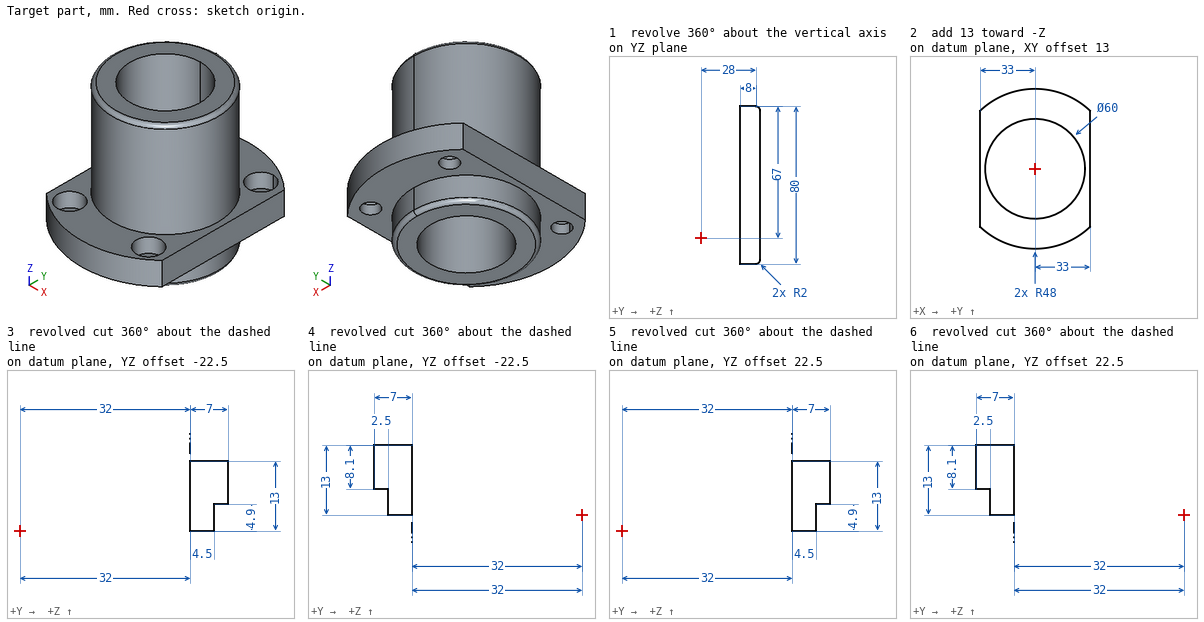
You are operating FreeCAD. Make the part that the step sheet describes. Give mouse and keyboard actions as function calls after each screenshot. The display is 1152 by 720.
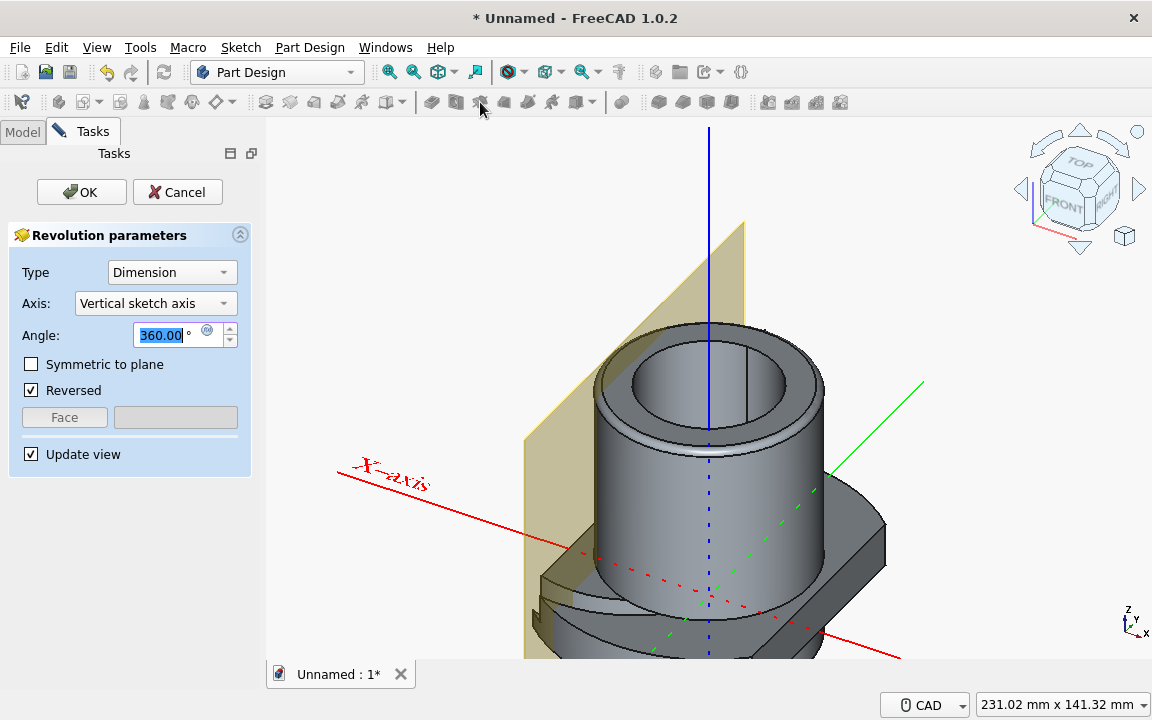
click(156, 304)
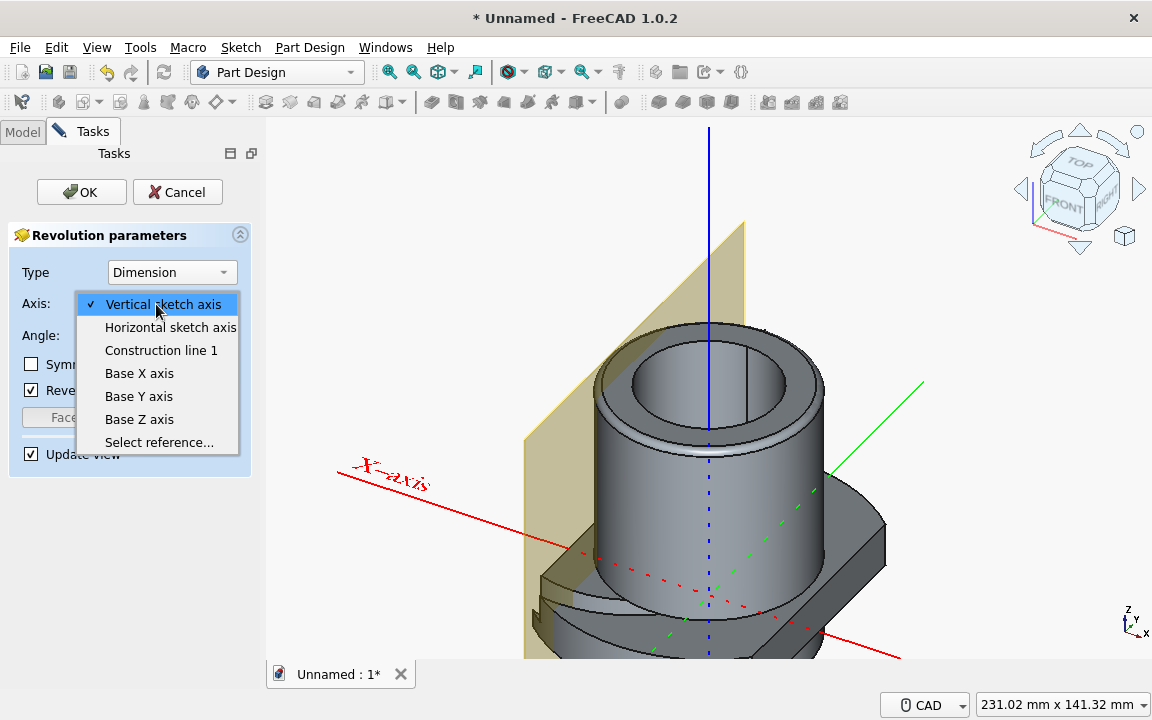
click(156, 350)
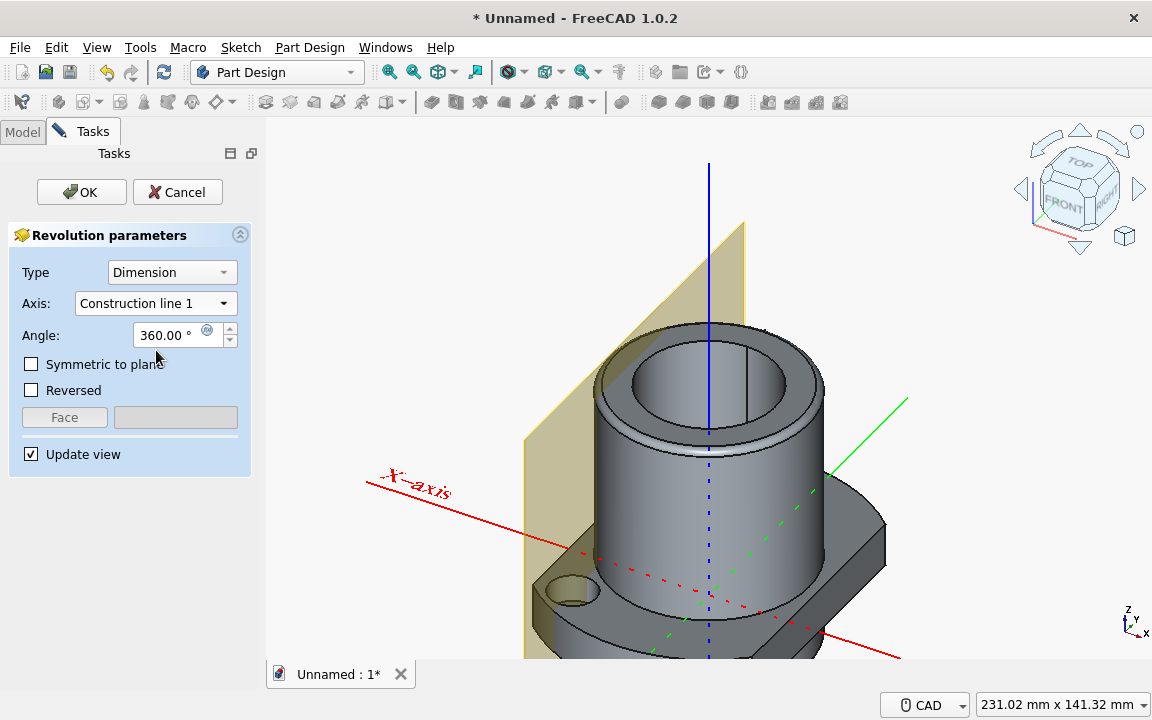
click(82, 192)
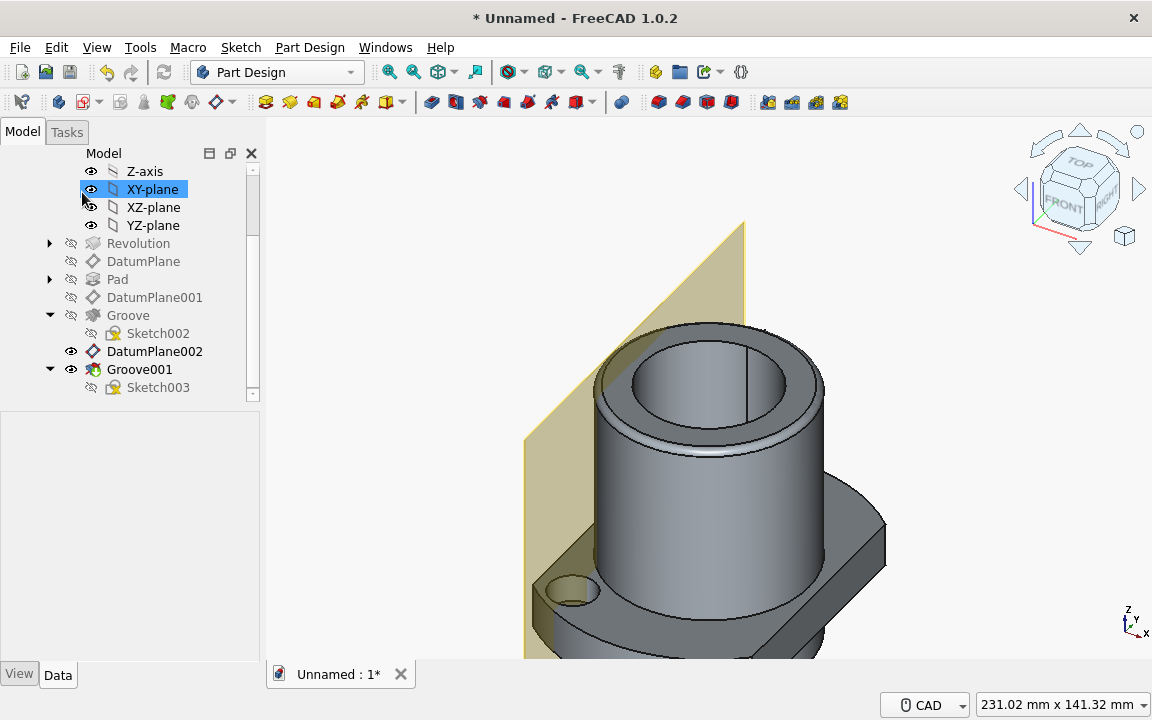
click(116, 351)
key(space)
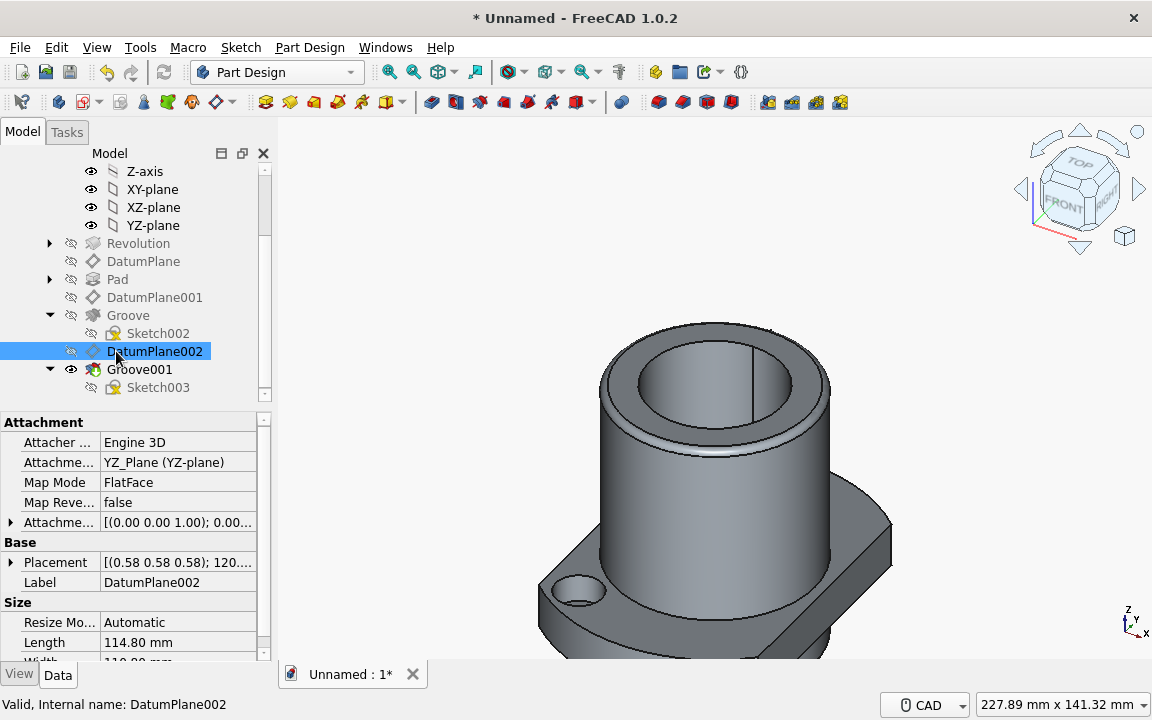
click(390, 72)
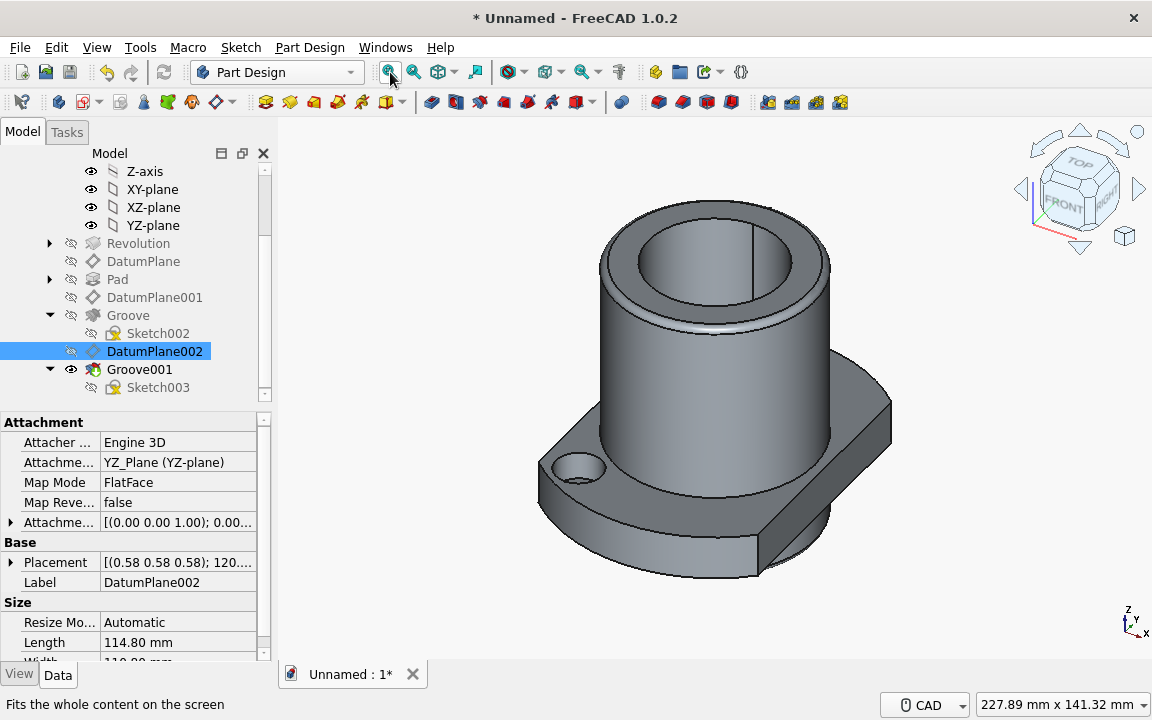
scroll(160, 275, down, 3)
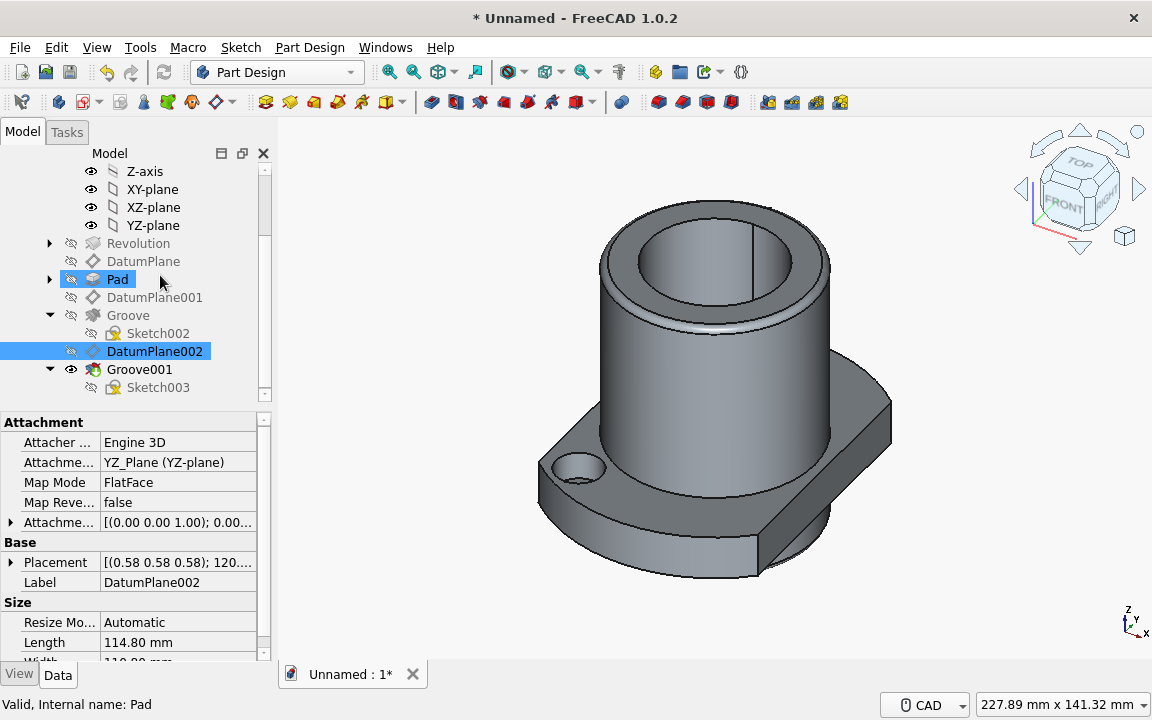
scroll(160, 275, up, 15)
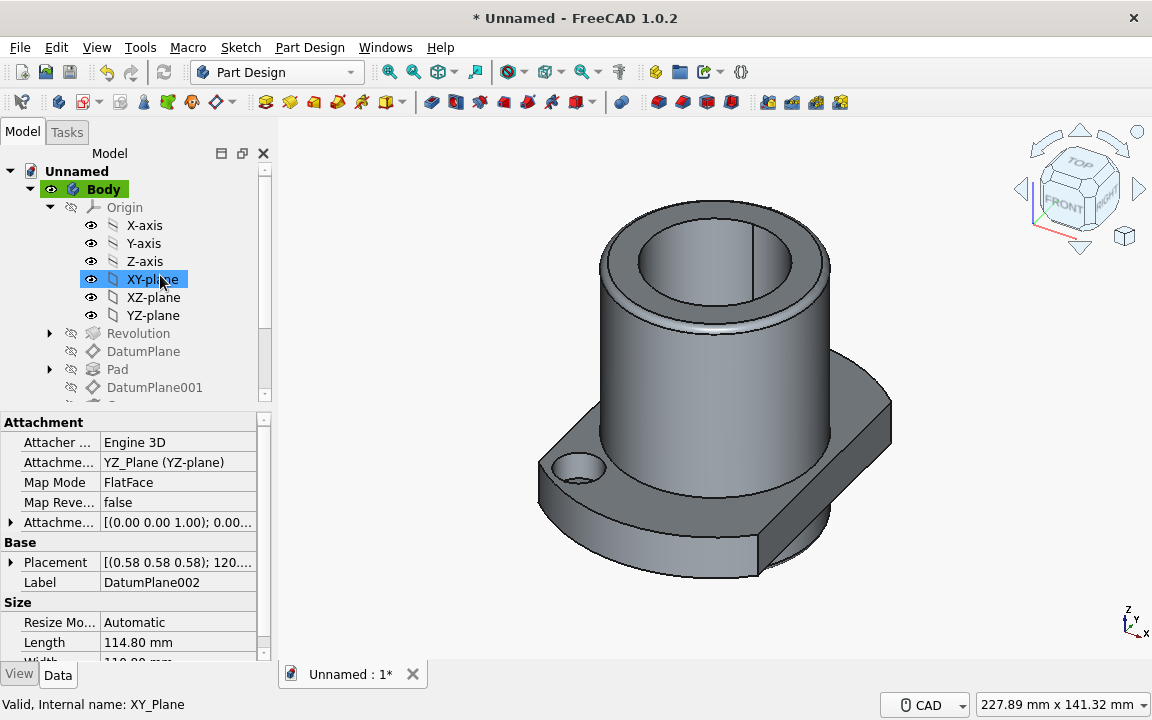
click(136, 315)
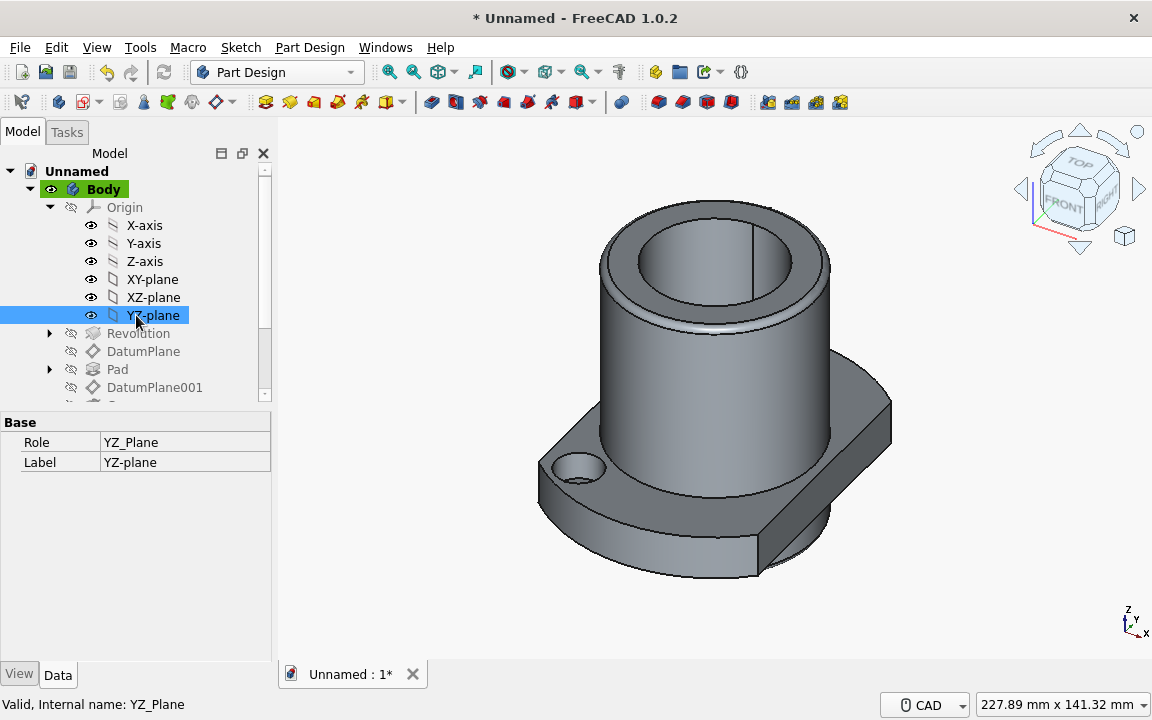
click(216, 102)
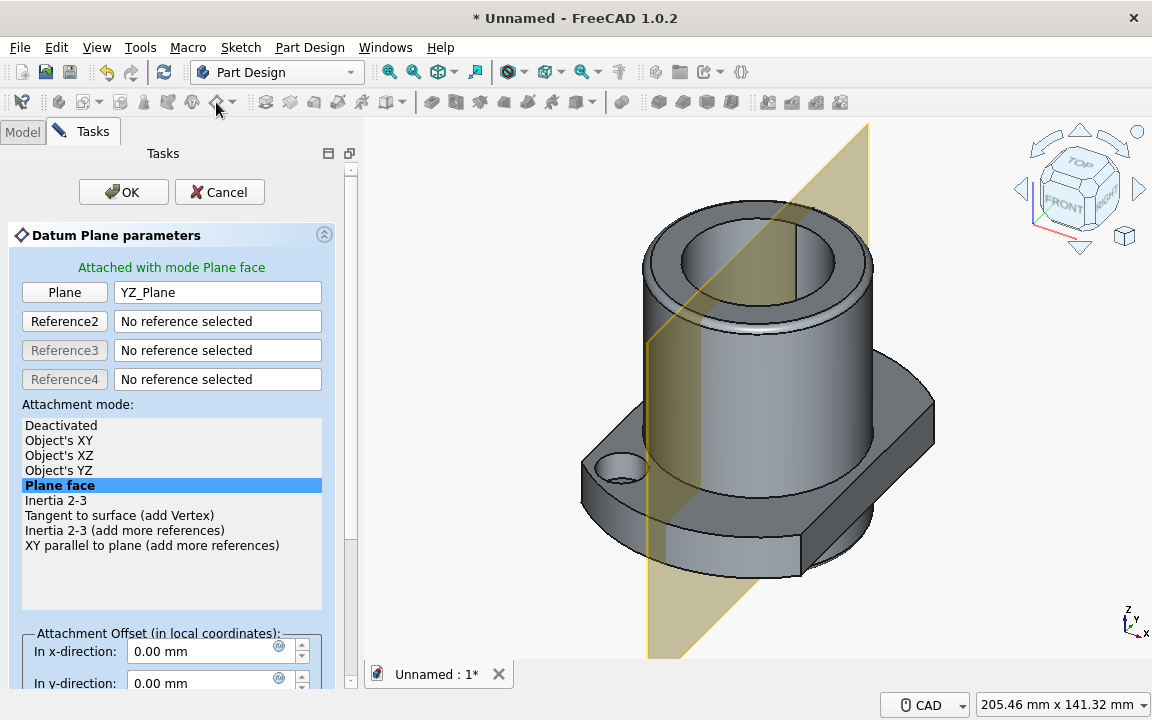
scroll(351, 426, down, 2)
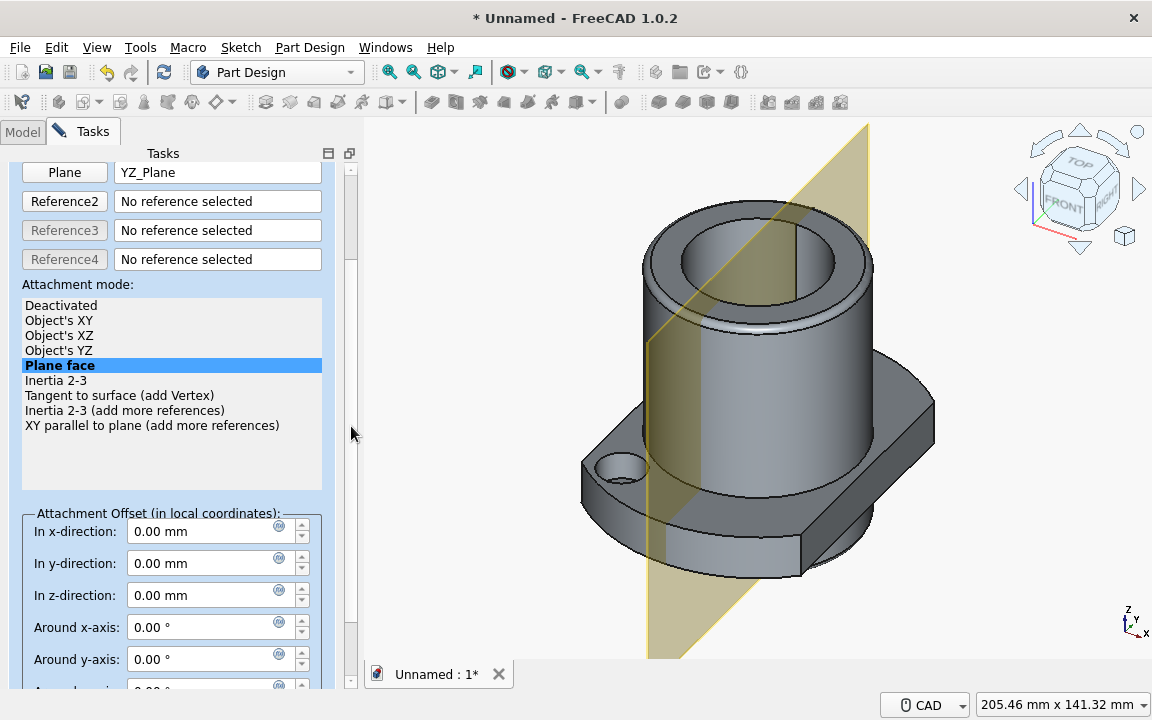
triple_click(210, 595)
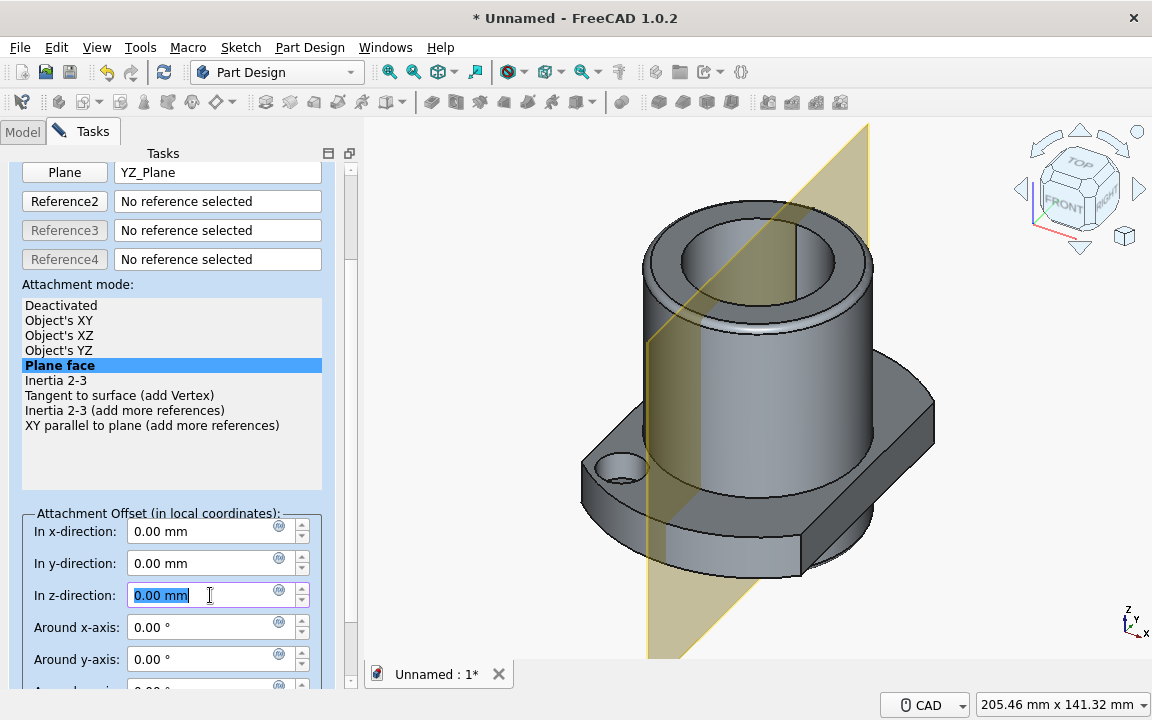
text(22.5)
key(Tab)